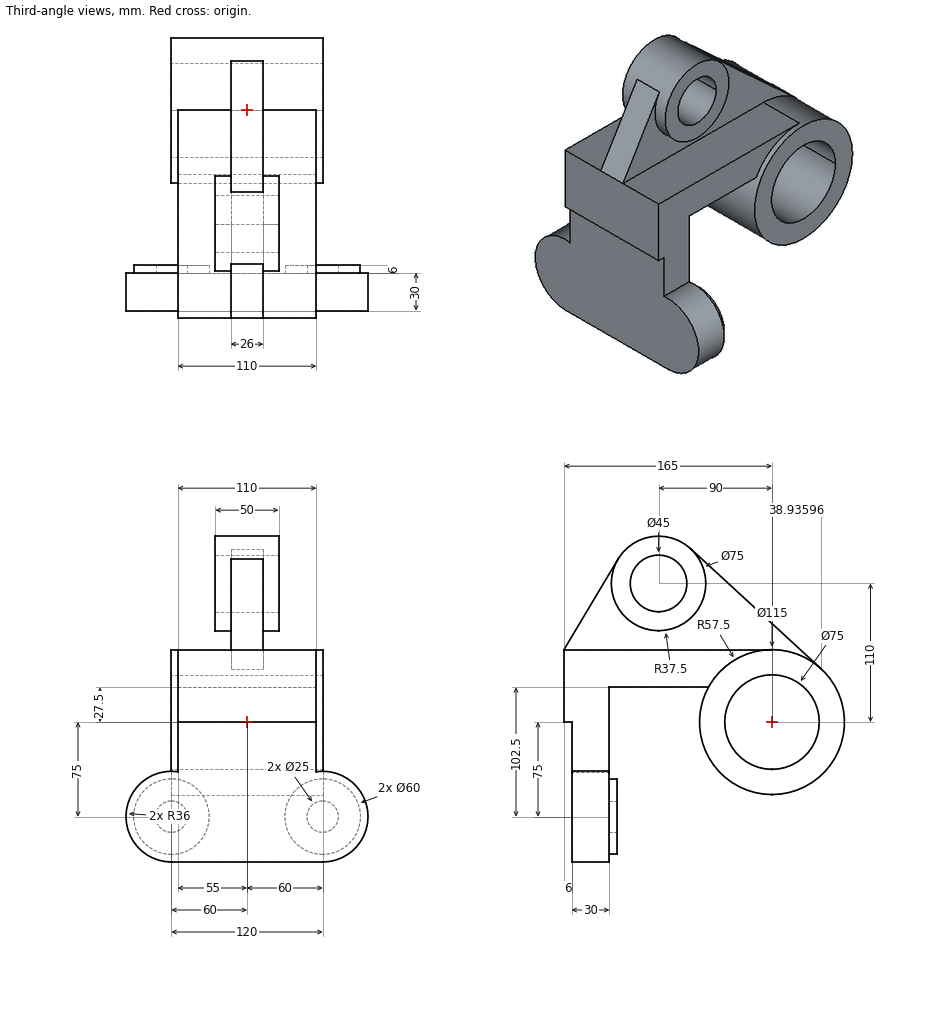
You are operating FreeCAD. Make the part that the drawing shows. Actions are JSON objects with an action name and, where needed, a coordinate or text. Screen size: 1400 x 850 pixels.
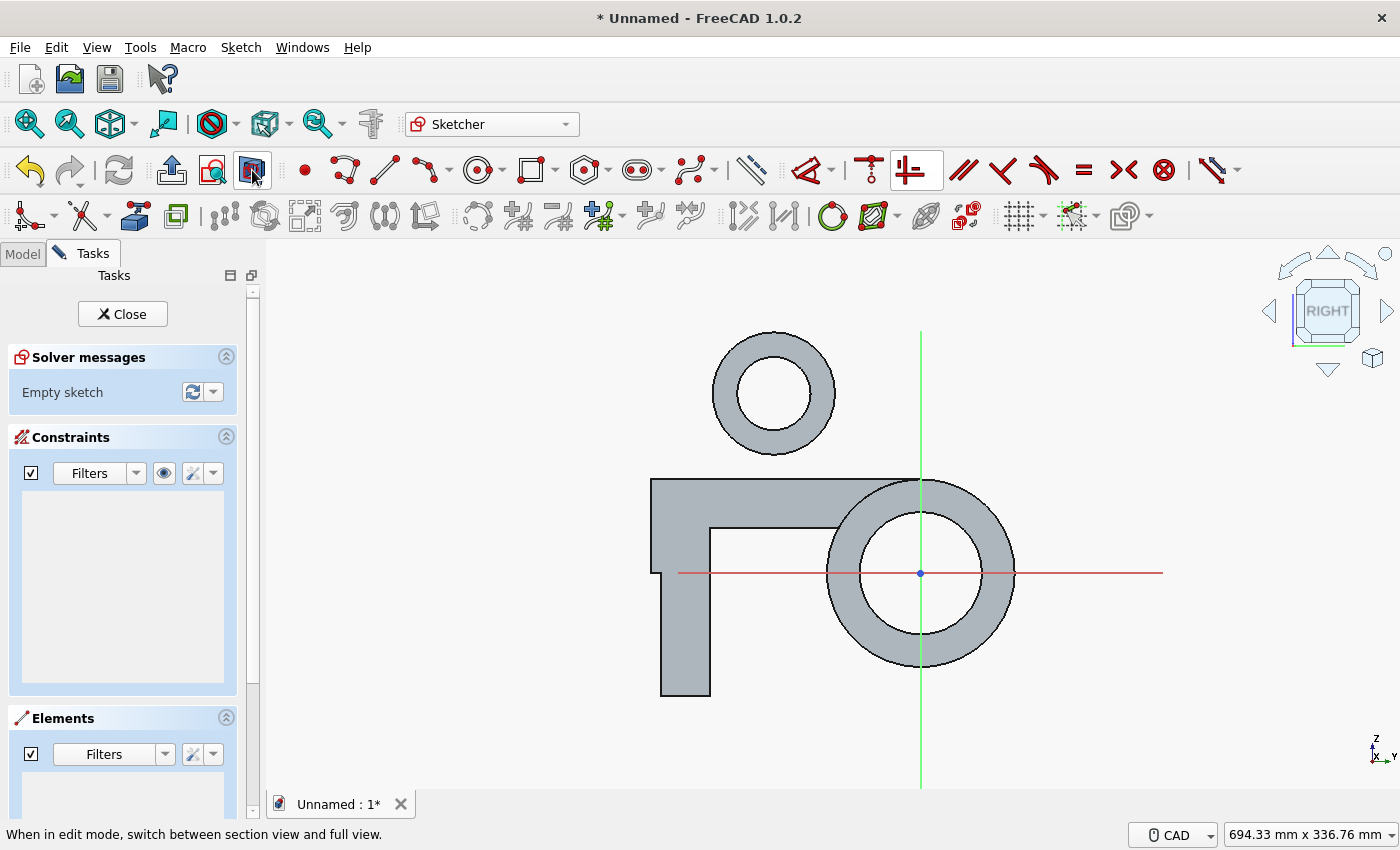
{"action": "scroll", "coordinate": [926, 353], "scroll_direction": "up", "scroll_amount": 2}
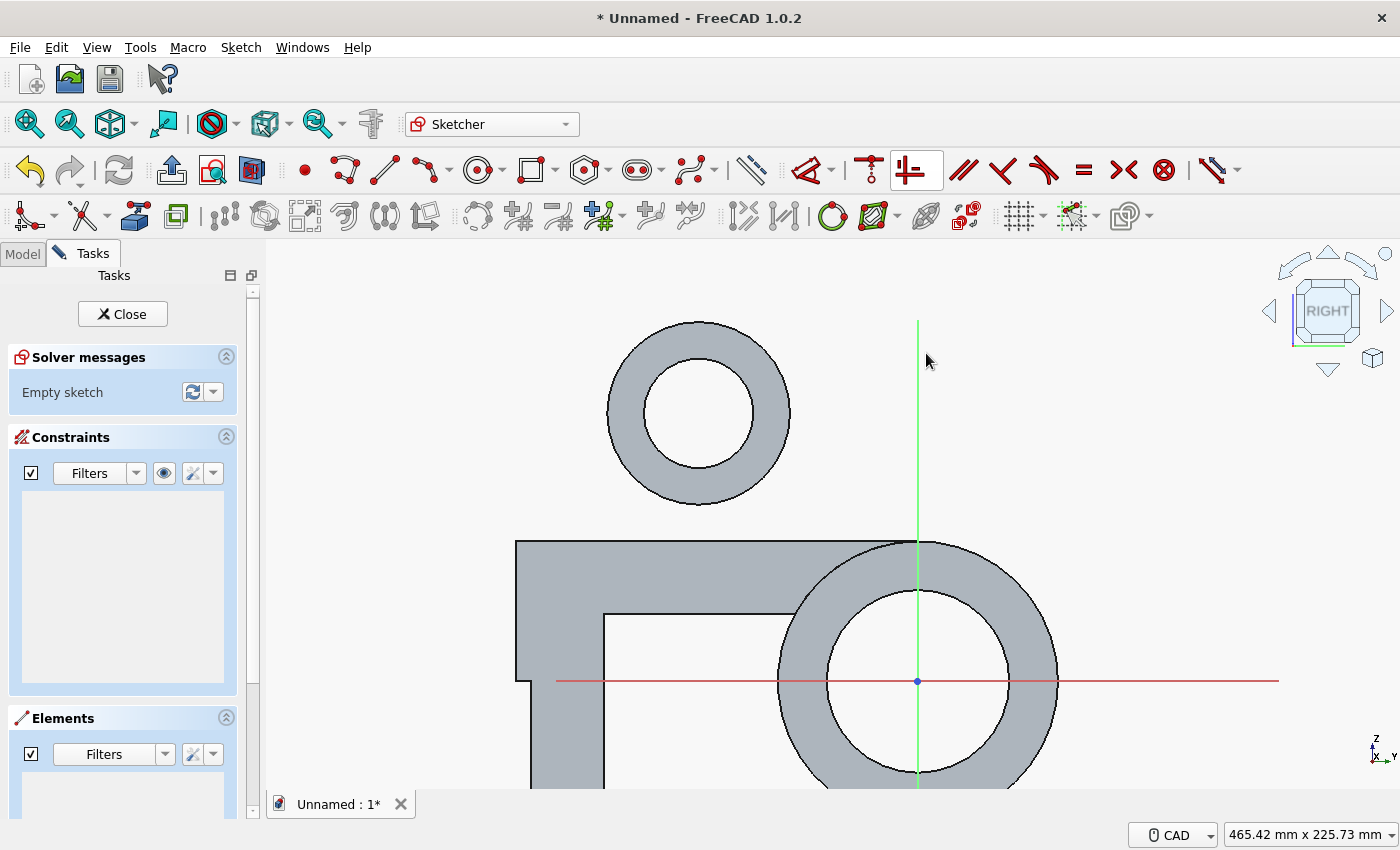
{"action": "left_click", "coordinate": [386, 170]}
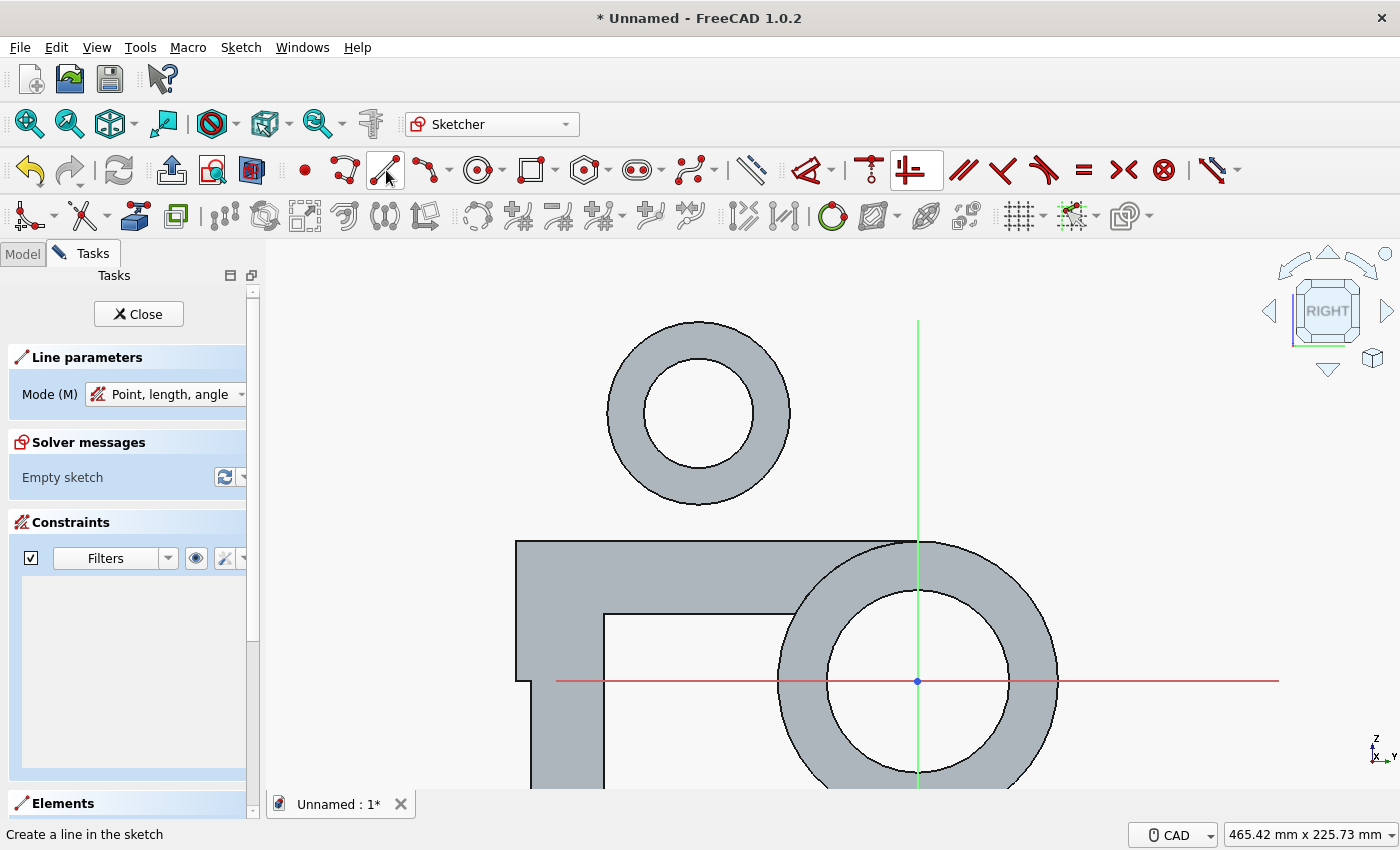
{"action": "left_click", "coordinate": [1013, 578]}
{"action": "left_click", "coordinate": [761, 346]}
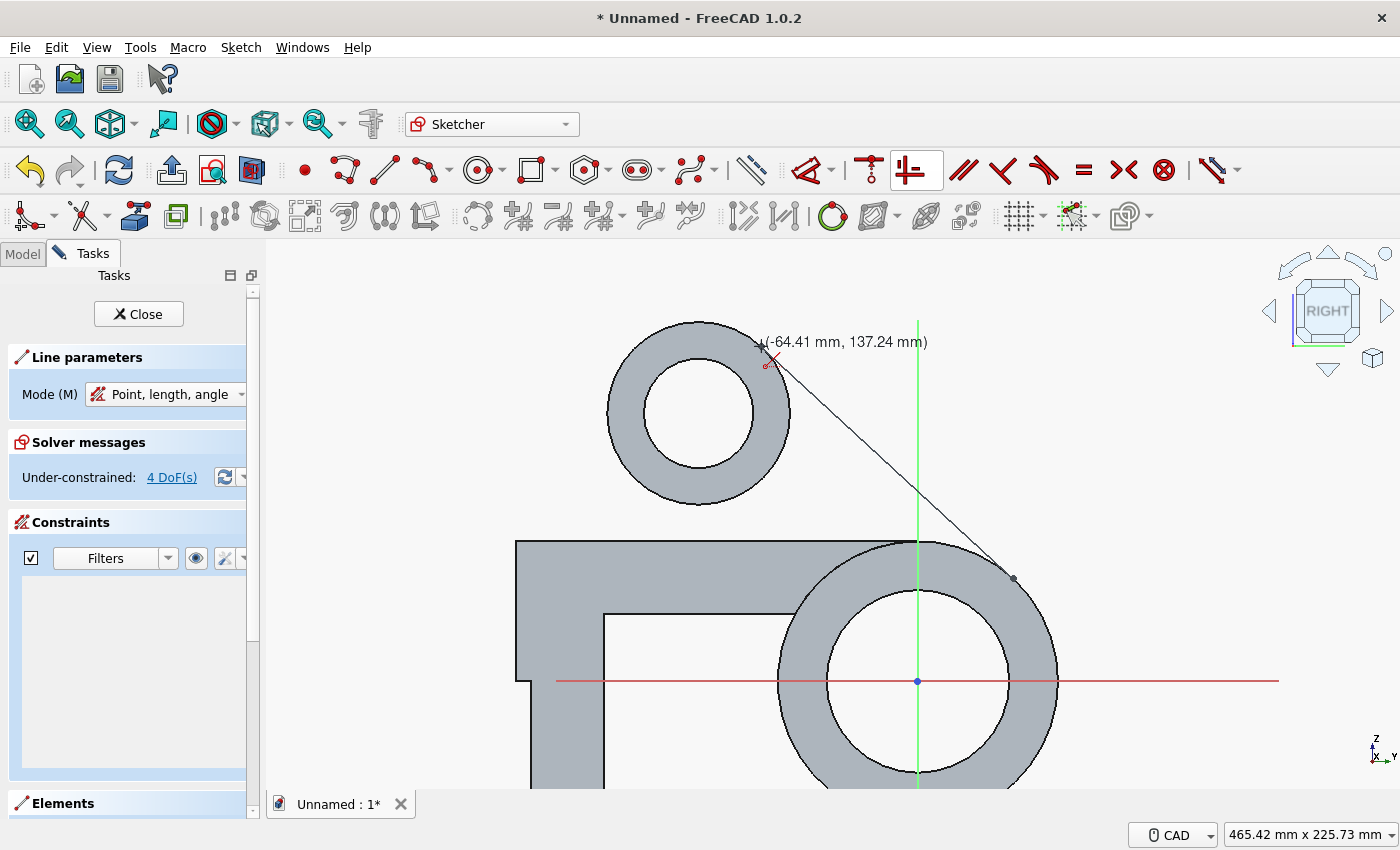
{"action": "left_click", "coordinate": [346, 170]}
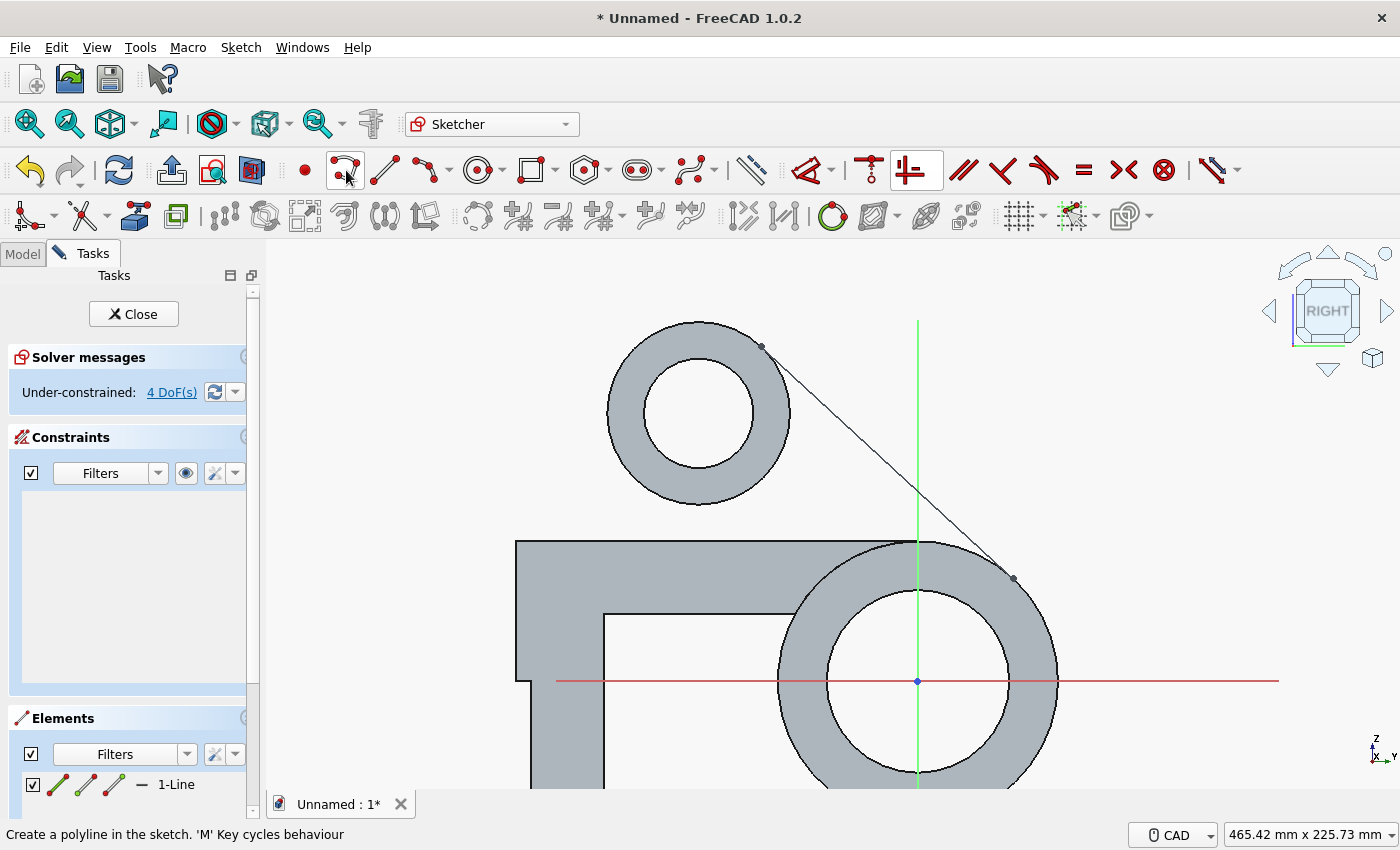
{"action": "left_click", "coordinate": [620, 367]}
{"action": "left_click", "coordinate": [516, 541]}
{"action": "left_click", "coordinate": [918, 541]}
{"action": "right_click", "coordinate": [918, 541]}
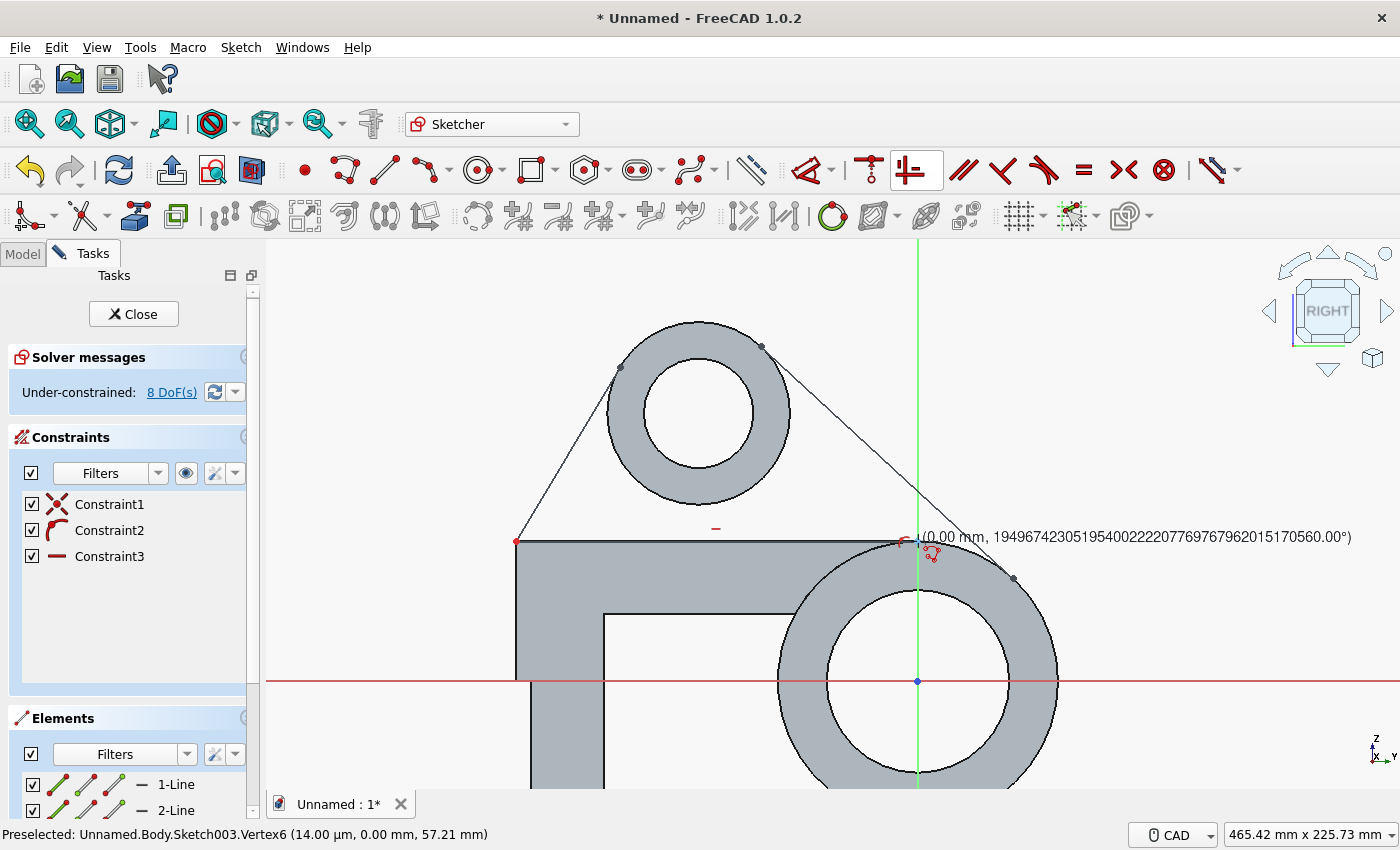
{"action": "left_click", "coordinate": [426, 170]}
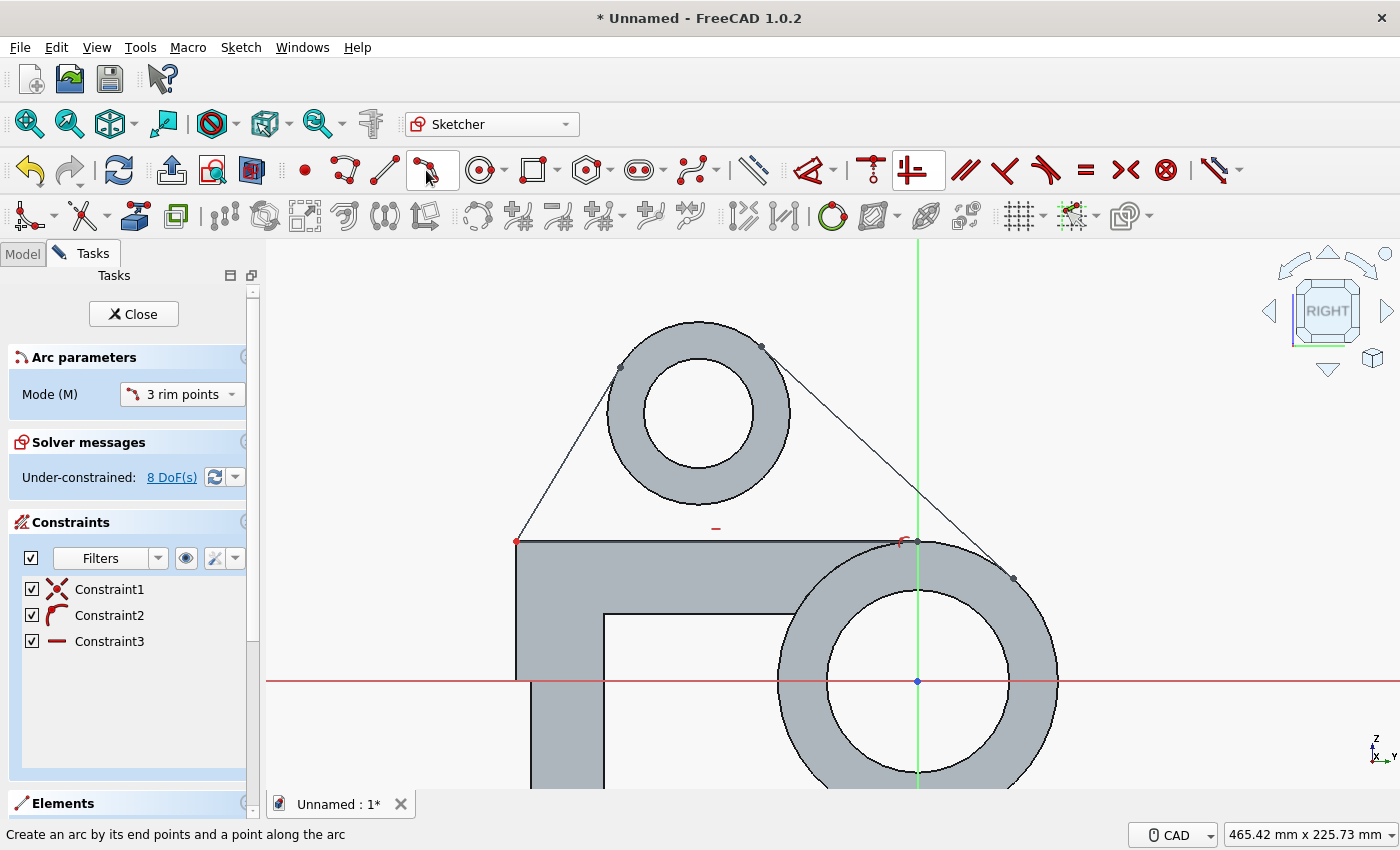
{"action": "left_click", "coordinate": [761, 347]}
{"action": "left_click", "coordinate": [620, 368]}
{"action": "left_click", "coordinate": [712, 504]}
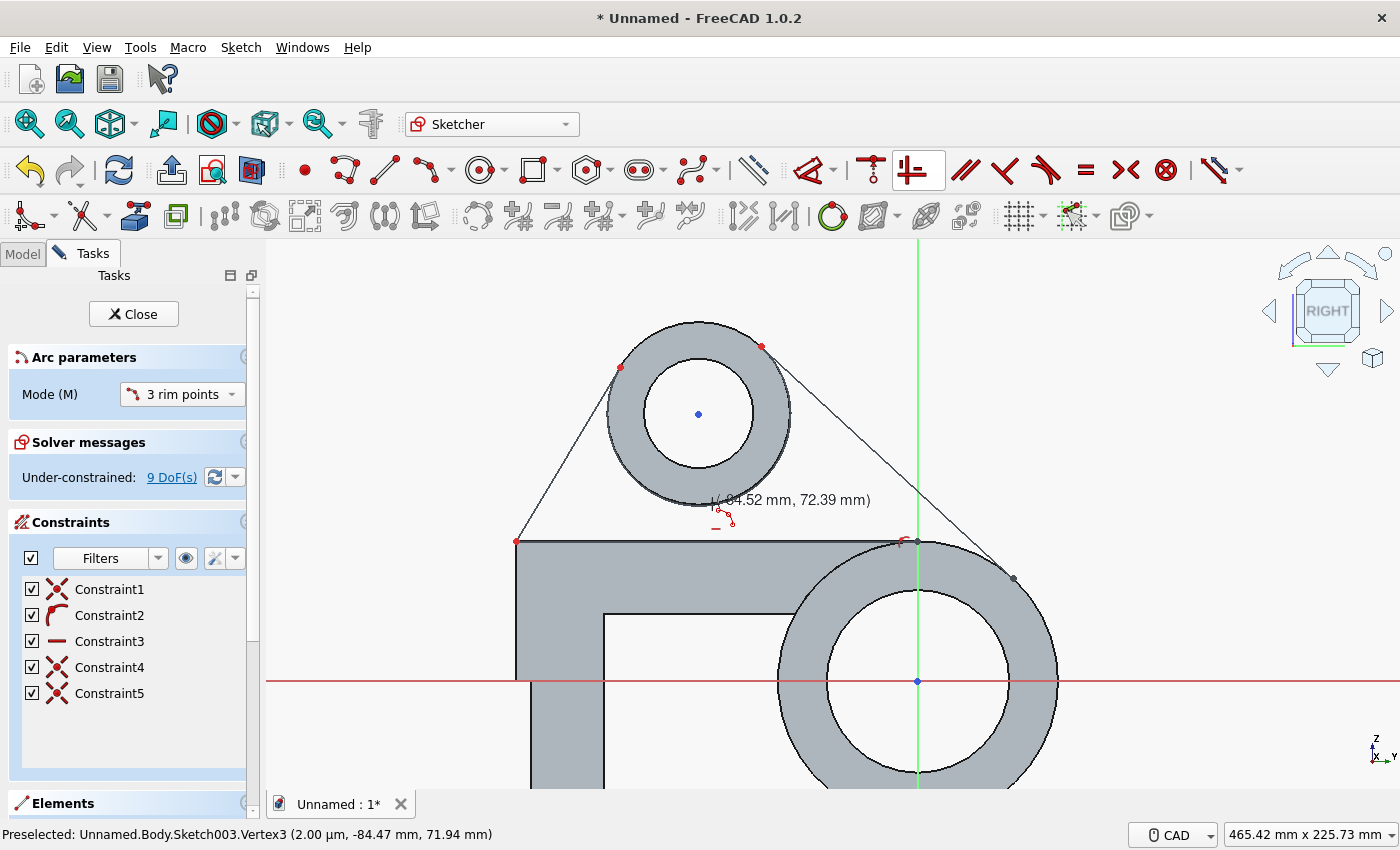
{"action": "left_click", "coordinate": [918, 542]}
{"action": "left_click", "coordinate": [1013, 579]}